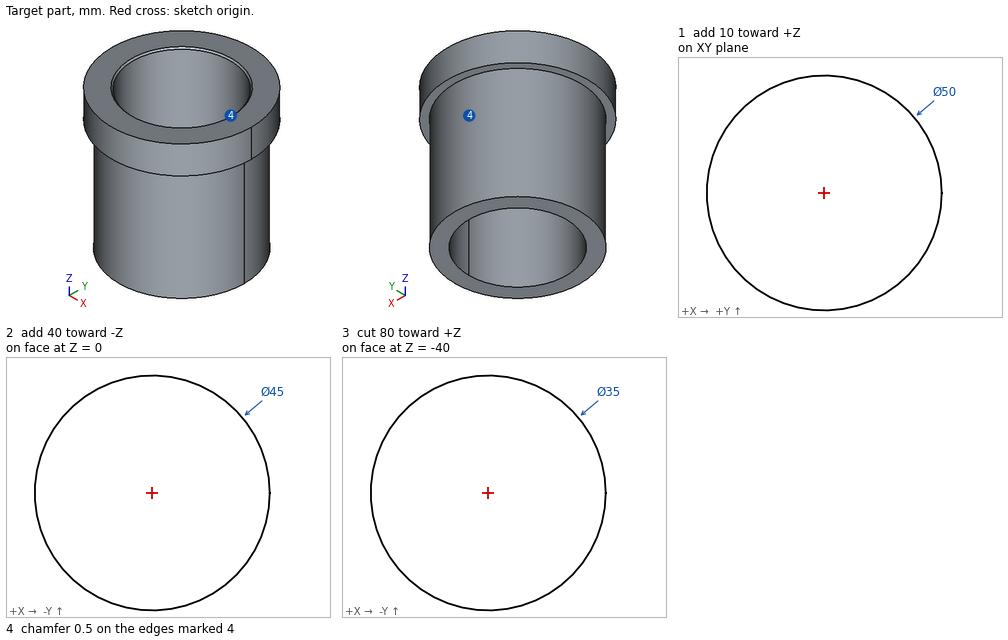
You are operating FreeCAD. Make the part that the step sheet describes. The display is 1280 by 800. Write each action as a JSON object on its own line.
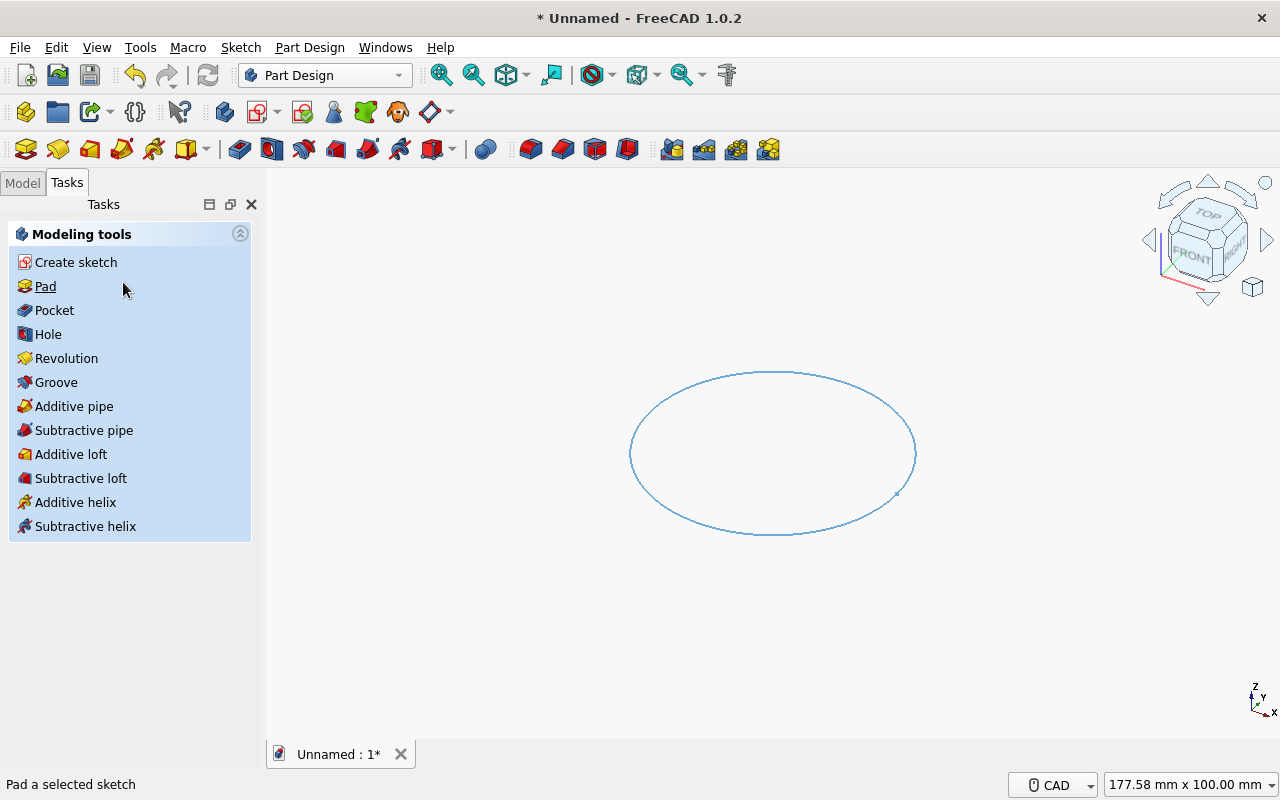
{"action": "left_click", "coordinate": [26, 150]}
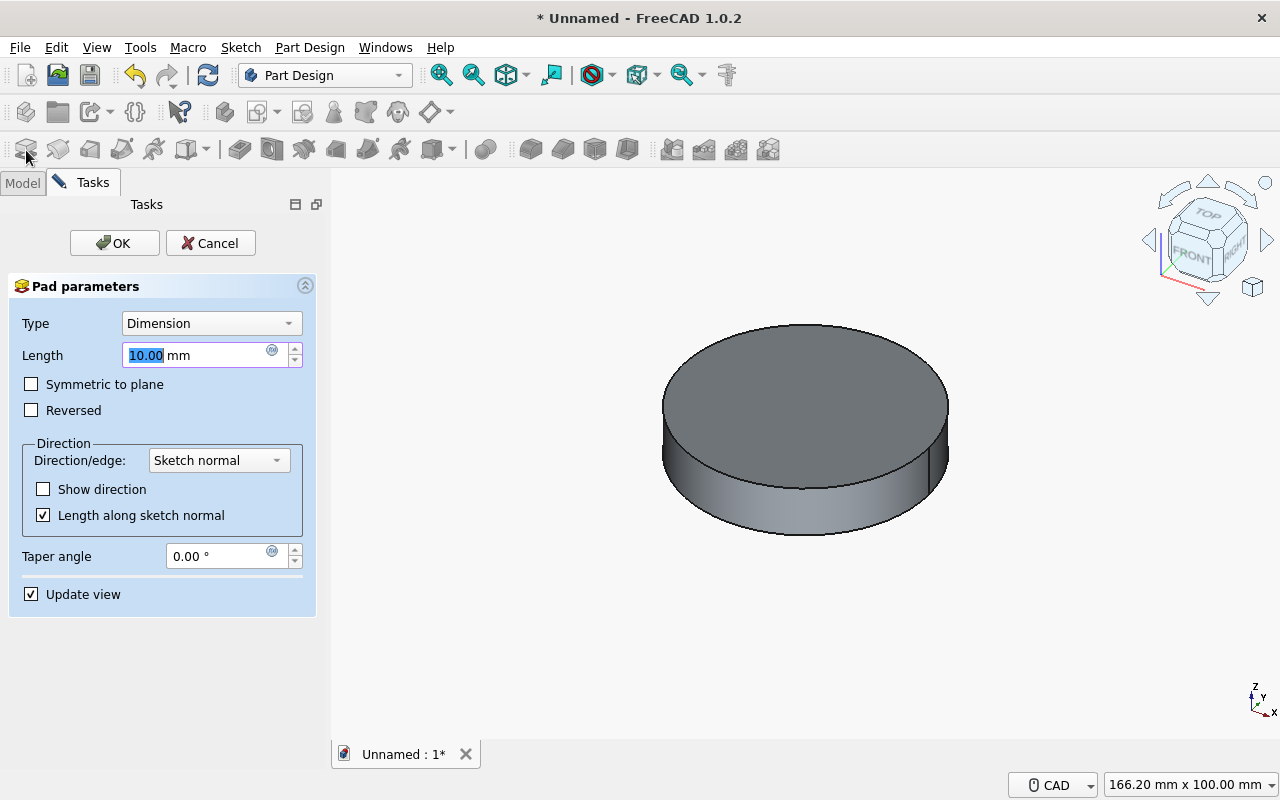
{"action": "type", "text": "10"}
{"action": "key", "text": "Tab"}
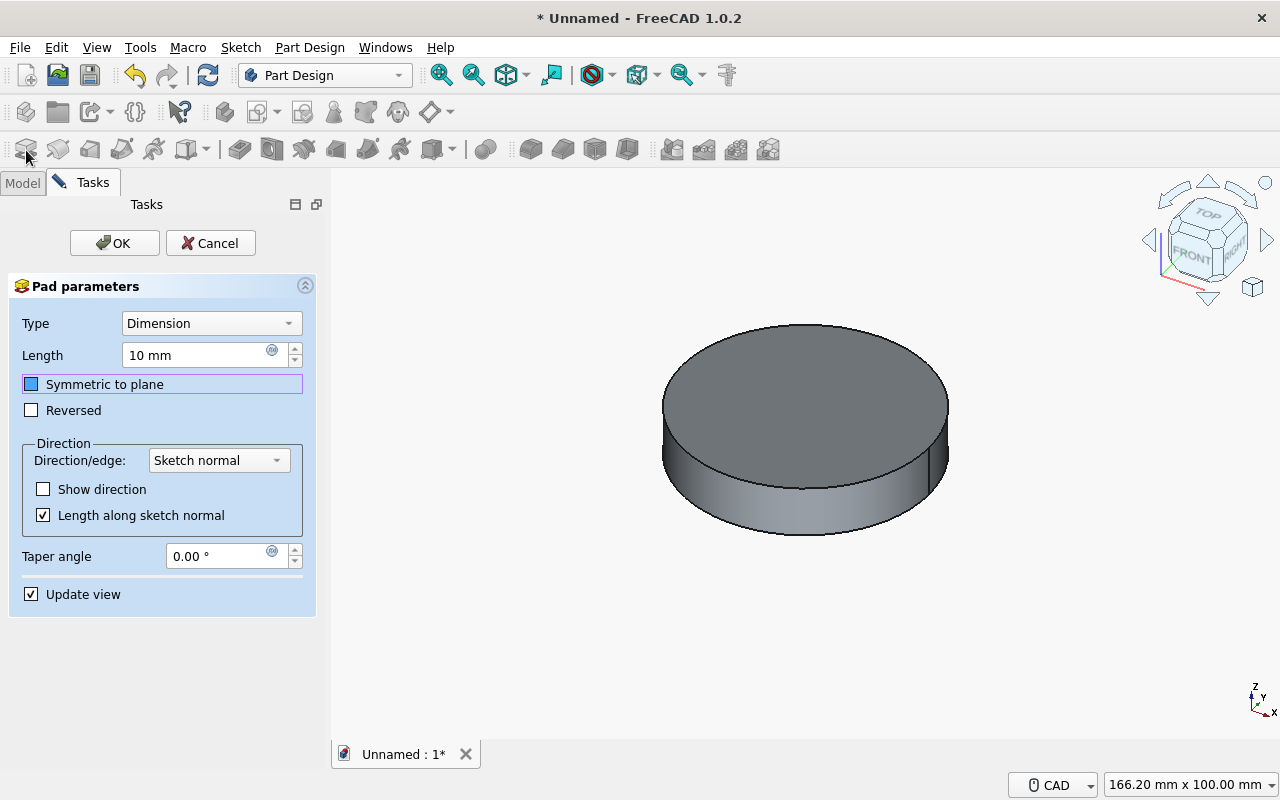
{"action": "left_click", "coordinate": [115, 243]}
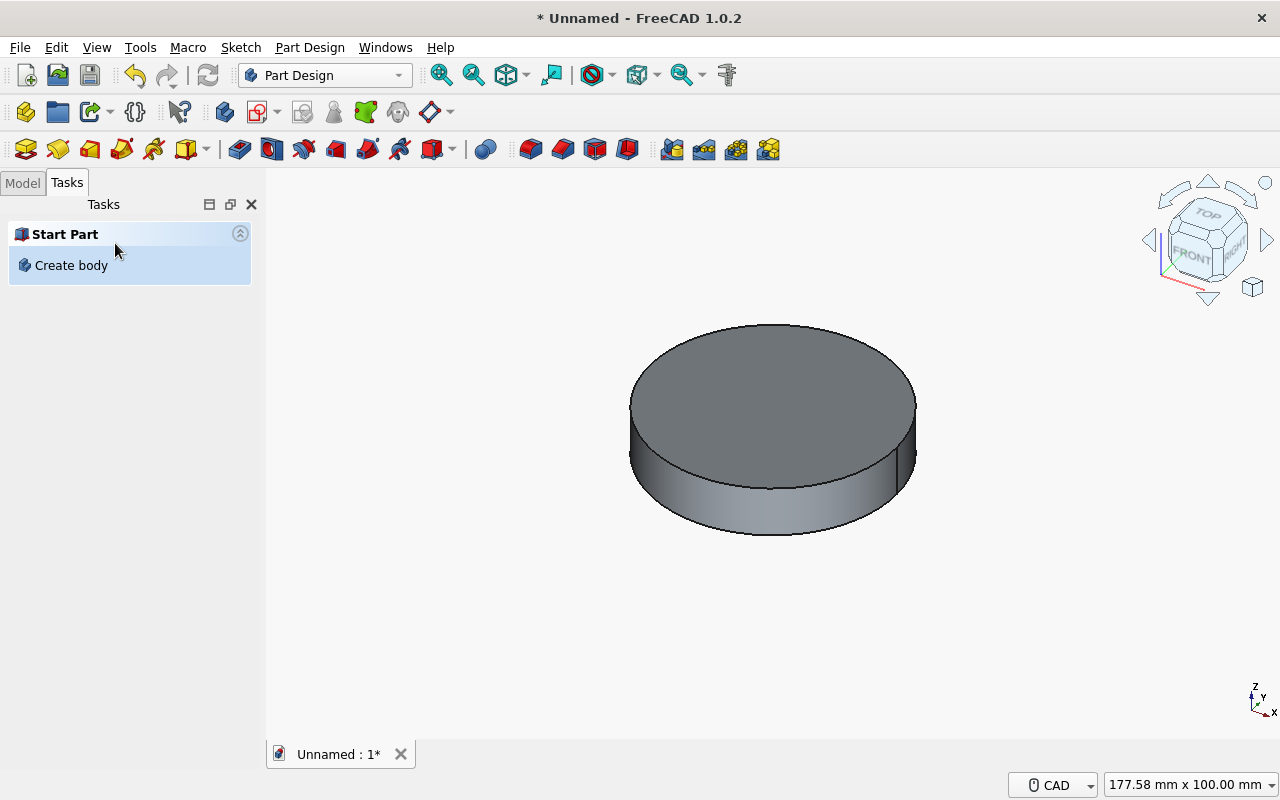
{"action": "key", "text": "5"}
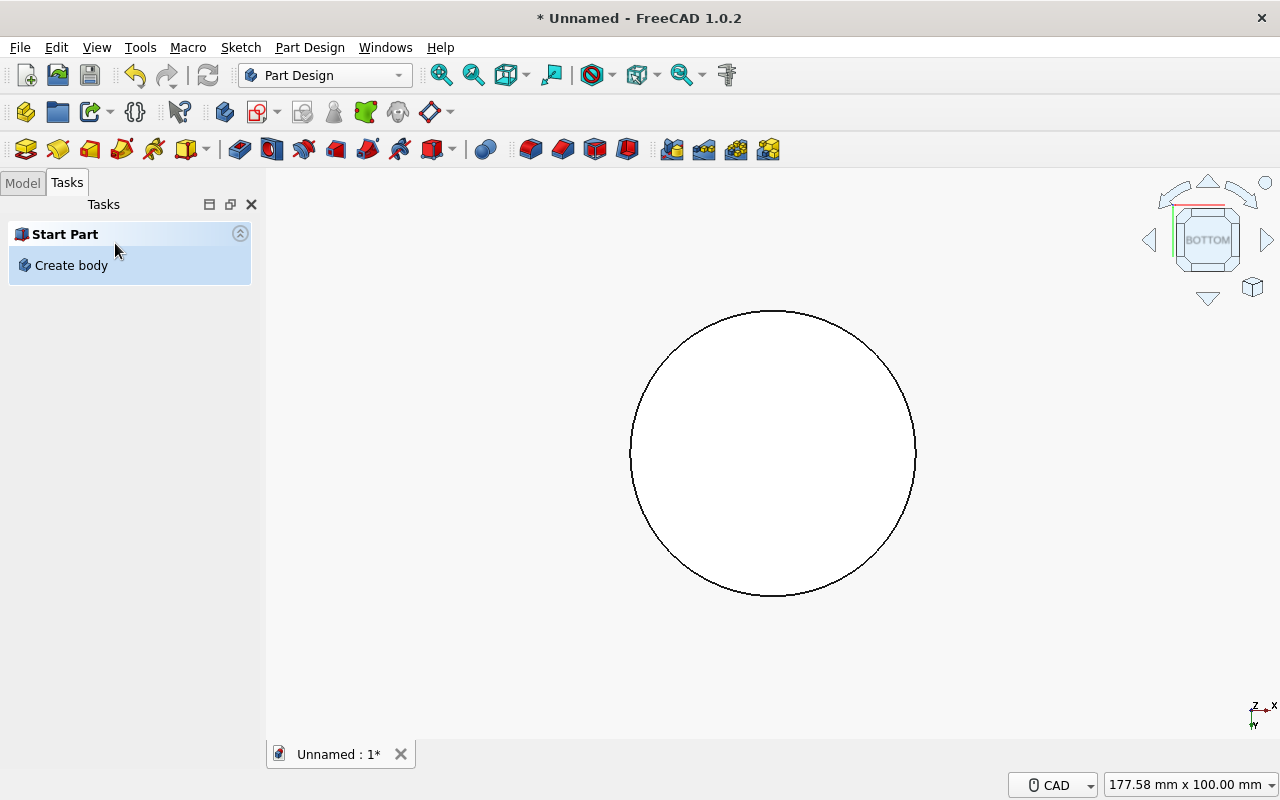
{"action": "left_click", "coordinate": [773, 452]}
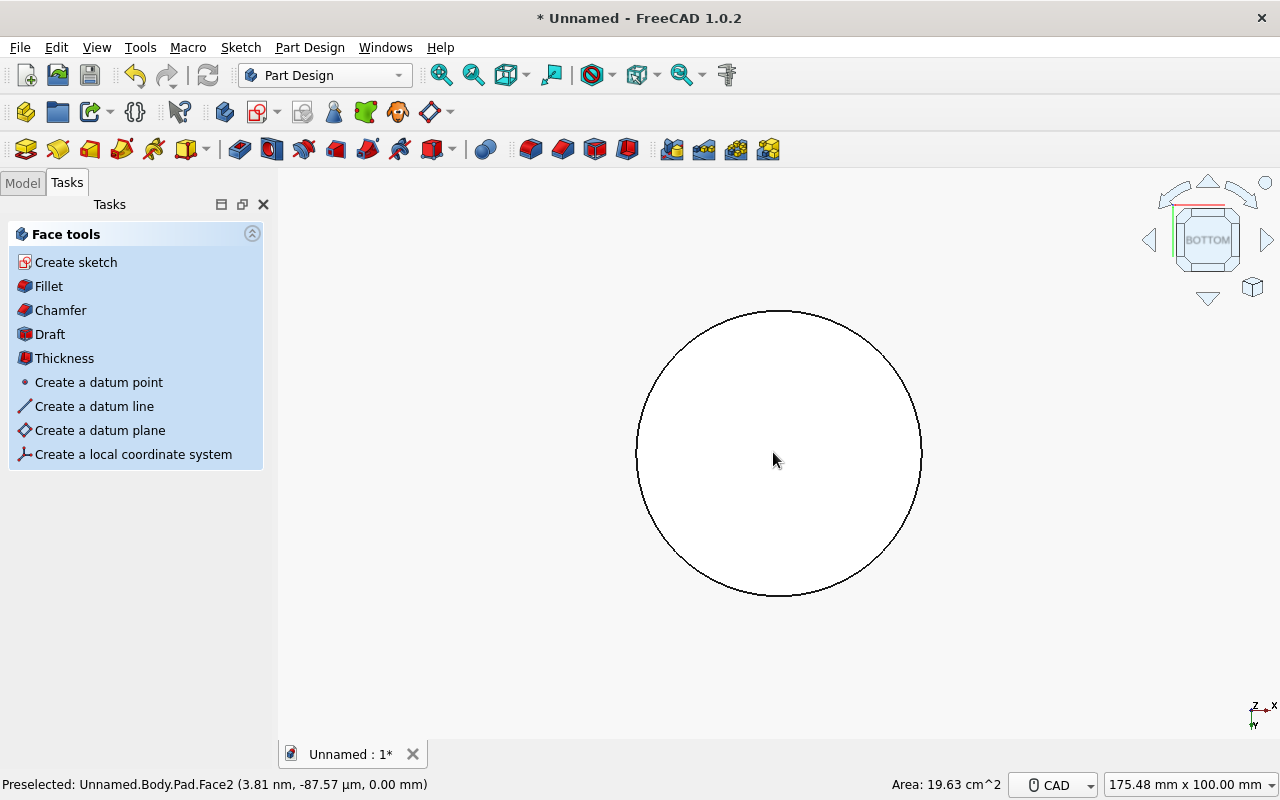
{"action": "left_click", "coordinate": [258, 112]}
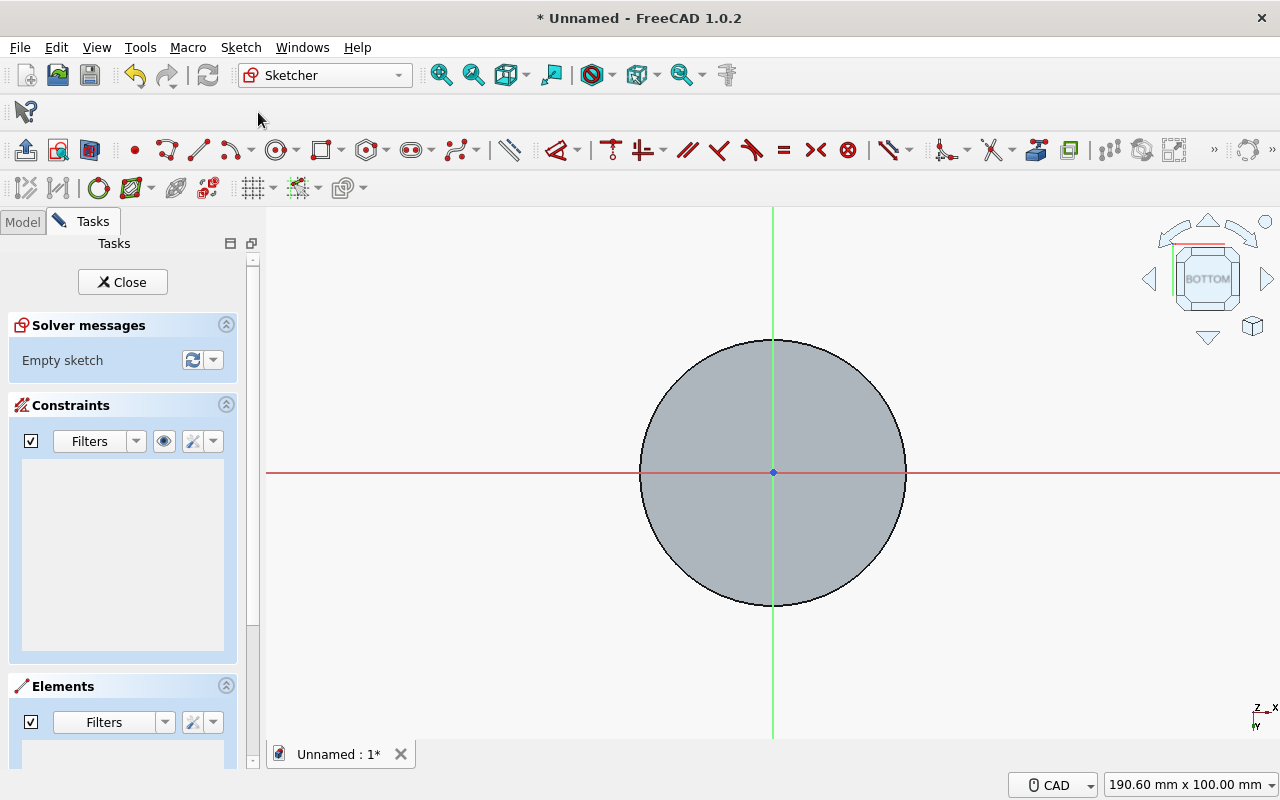
{"action": "scroll", "coordinate": [912, 473], "scroll_direction": "up", "scroll_amount": 2}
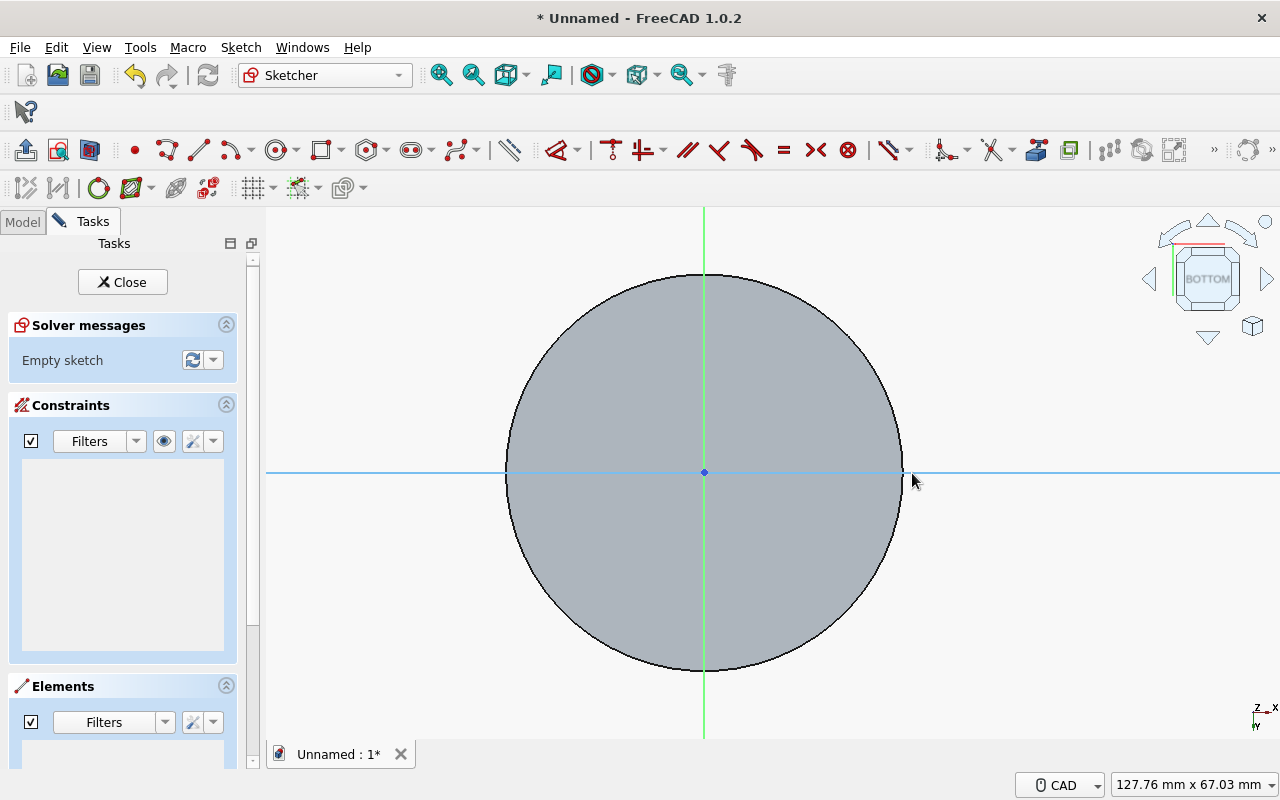
{"action": "key", "text": "g c"}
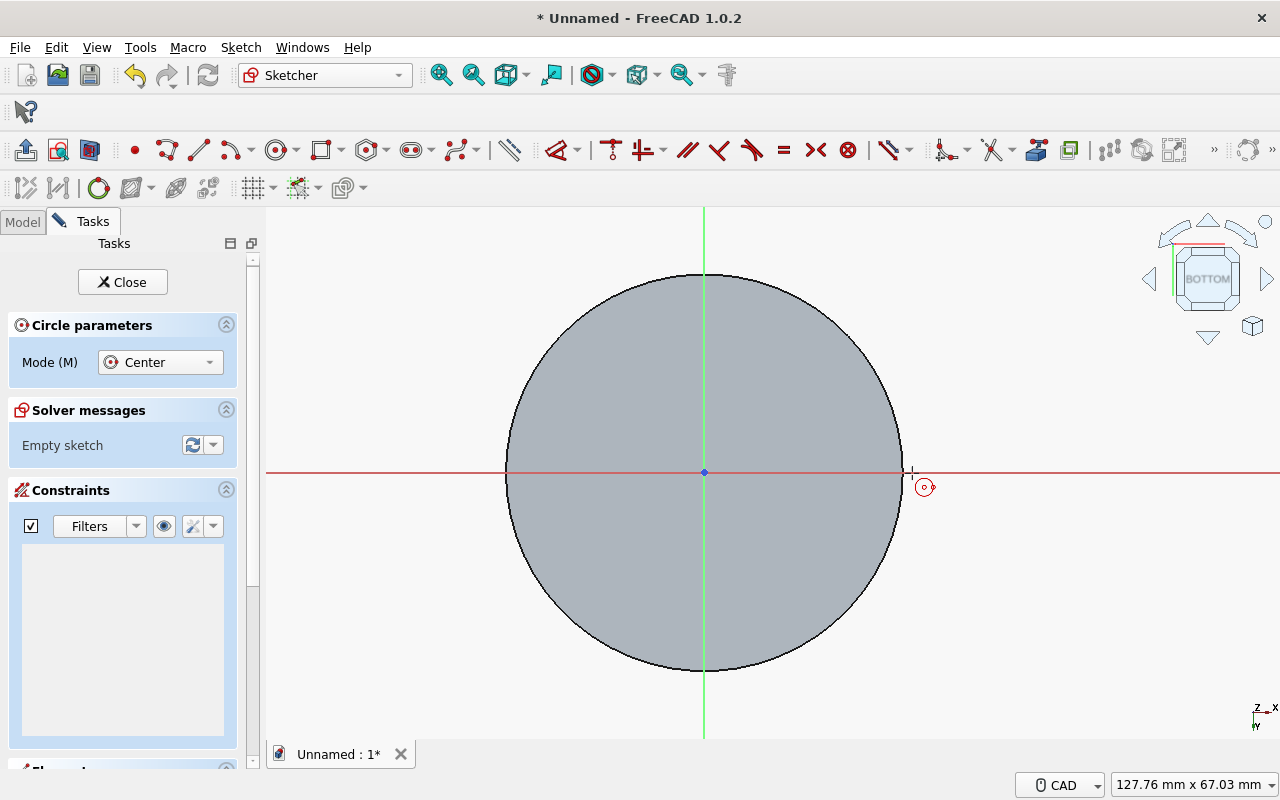
{"action": "left_click", "coordinate": [704, 473]}
{"action": "left_click", "coordinate": [831, 346]}
{"action": "key", "text": "Escape"}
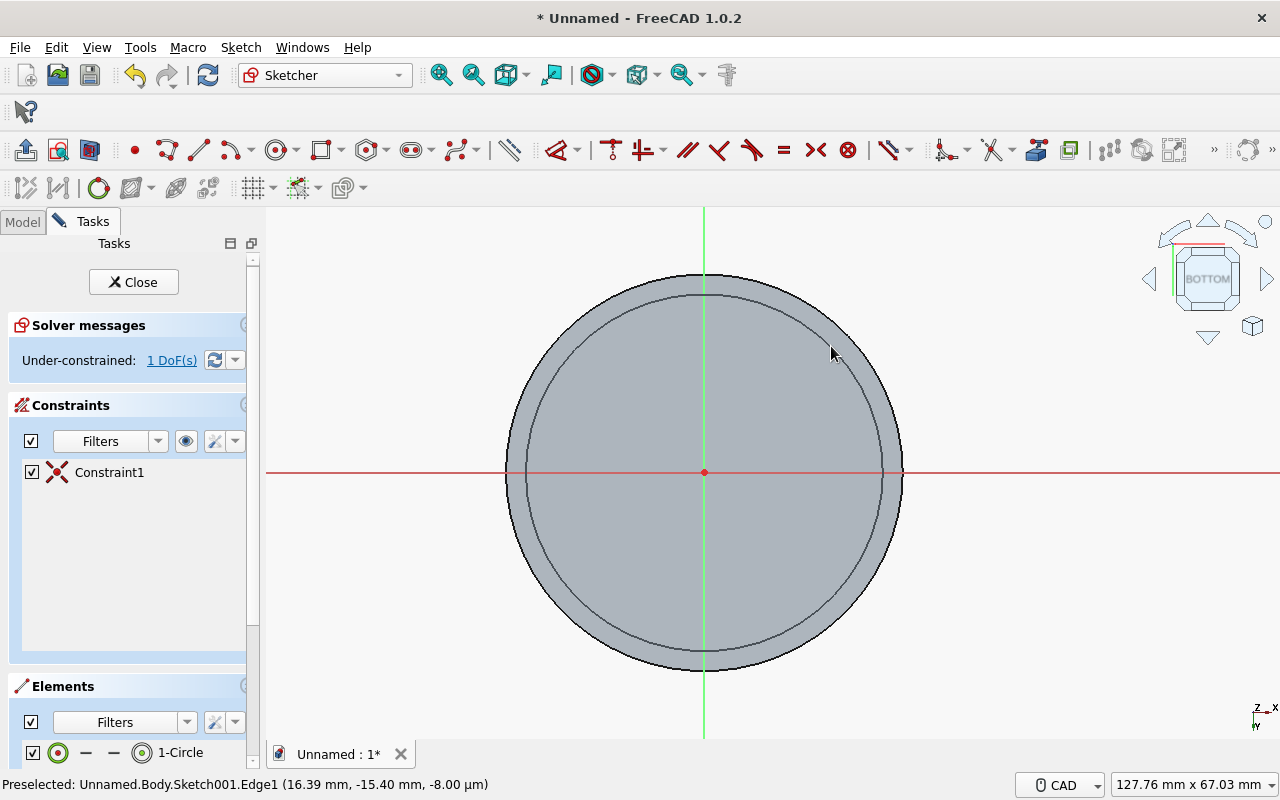
{"action": "left_click", "coordinate": [556, 150]}